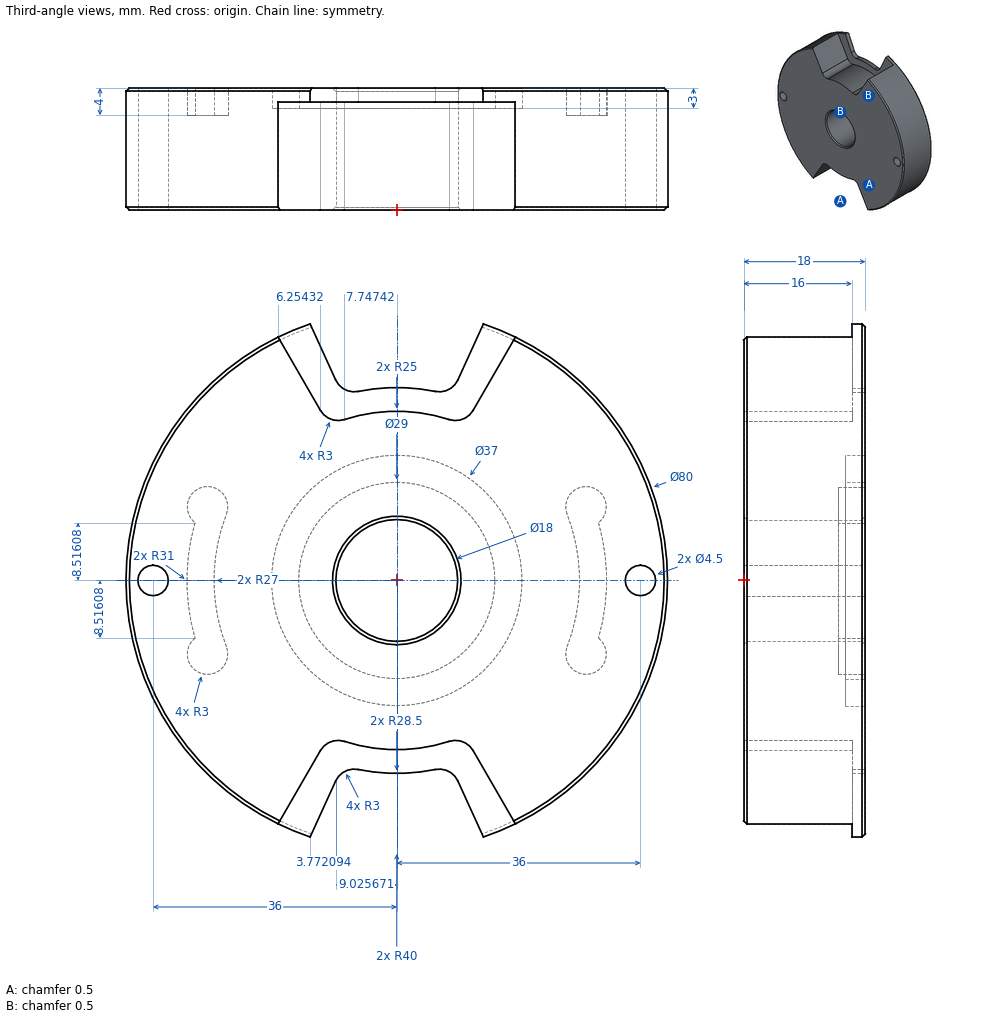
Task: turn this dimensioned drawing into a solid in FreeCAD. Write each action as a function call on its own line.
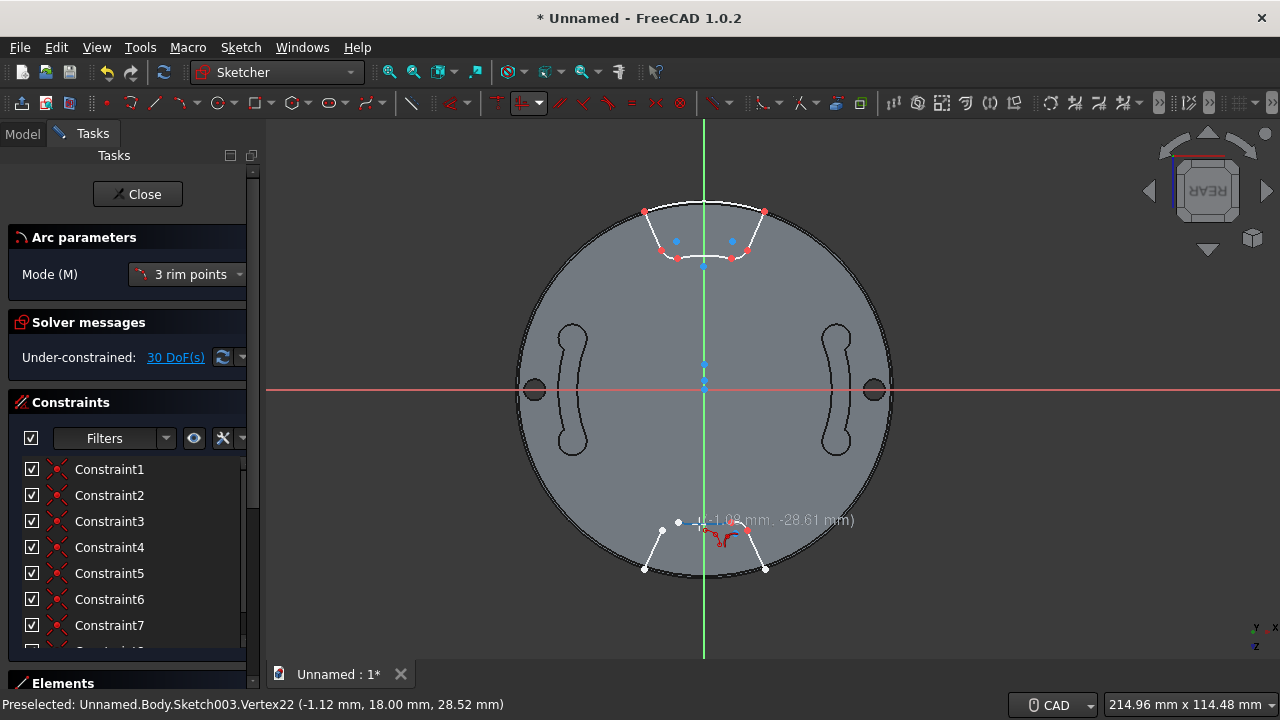
click(678, 523)
click(662, 531)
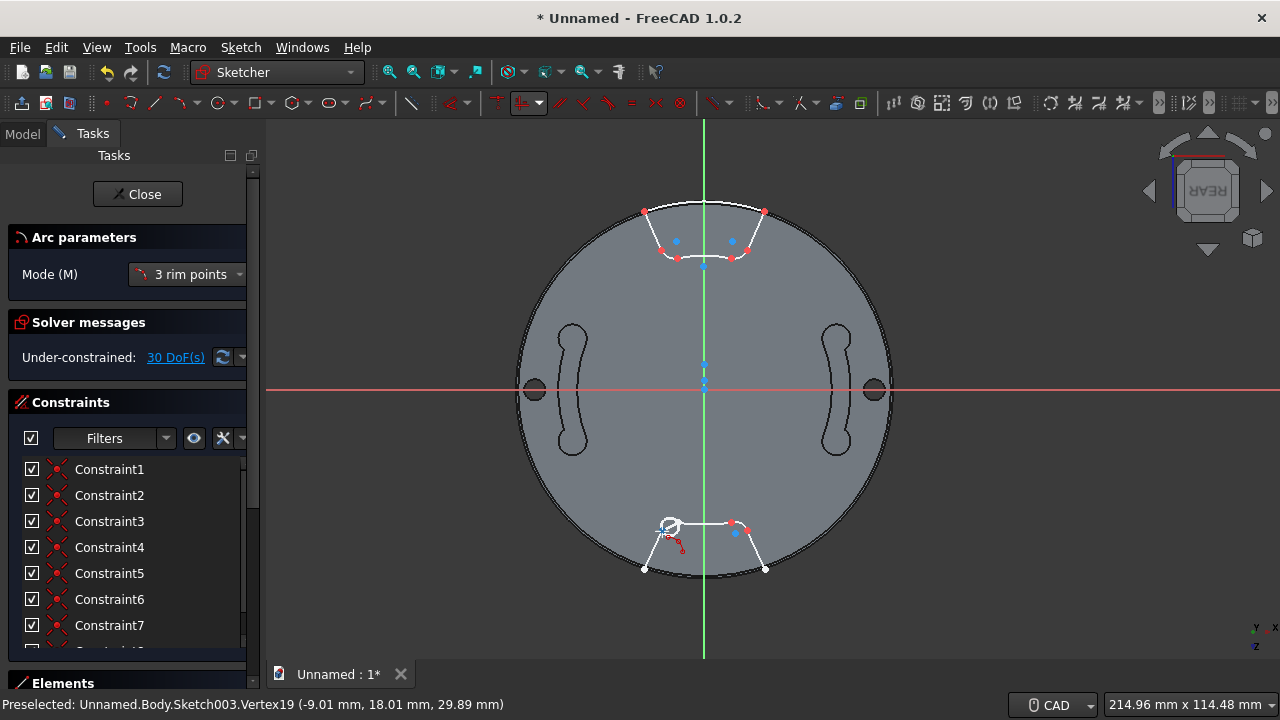
scroll(668, 523, up, 9)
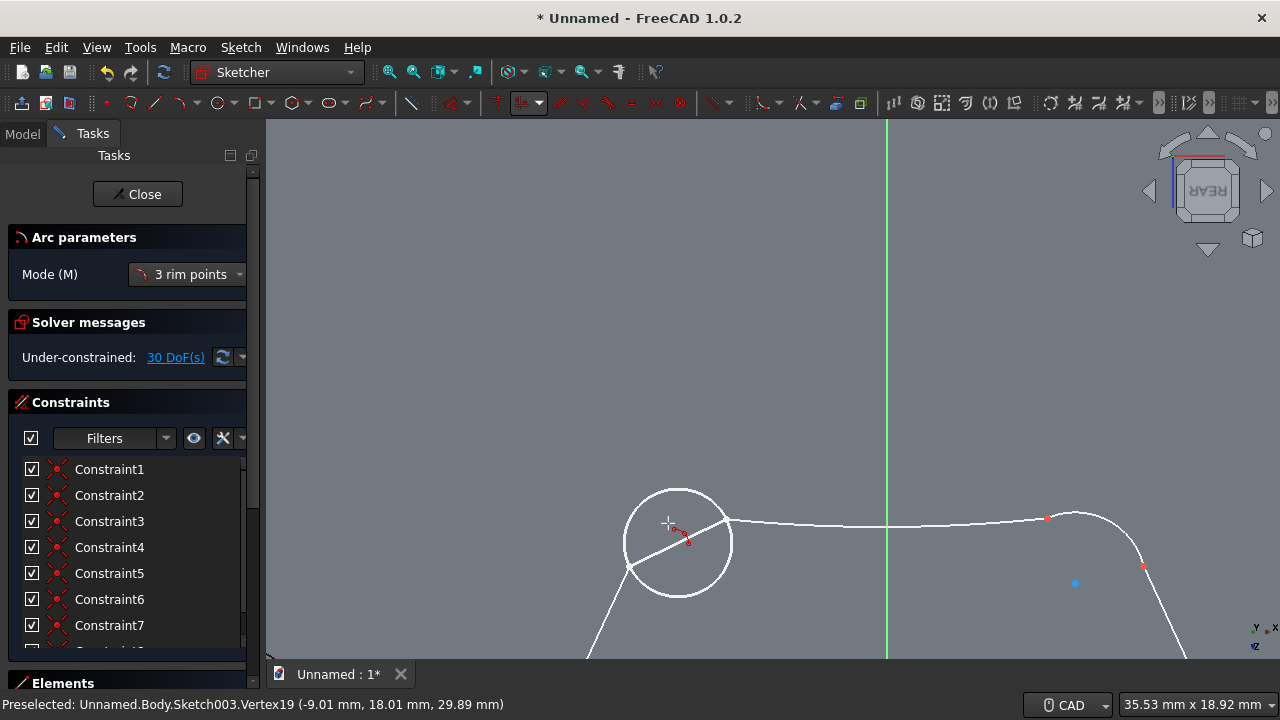
click(668, 518)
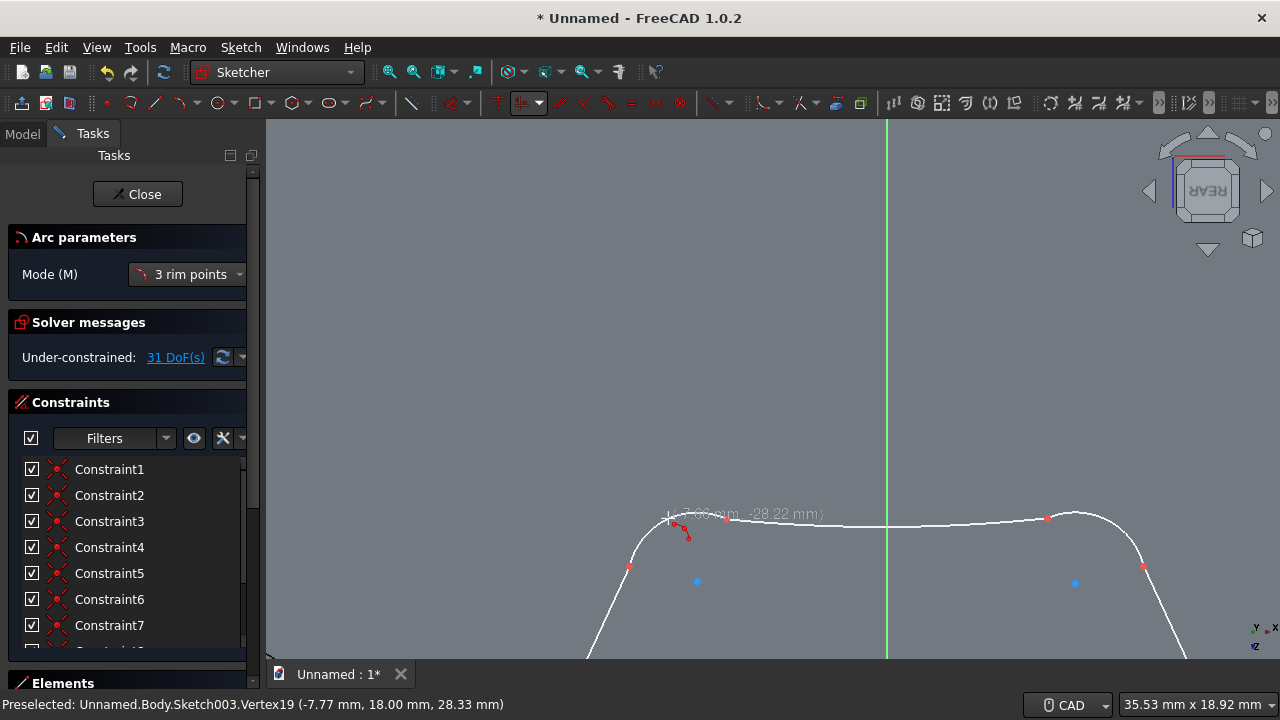
scroll(668, 523, down, 9)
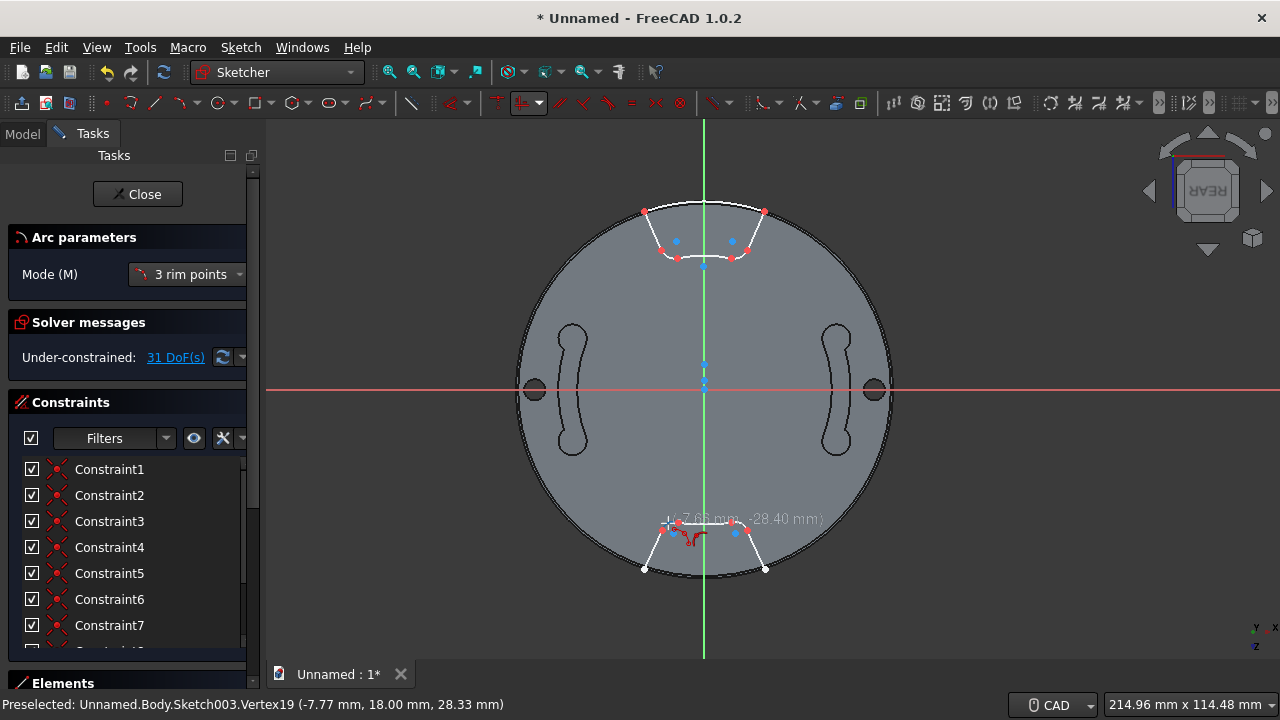
click(644, 570)
click(765, 570)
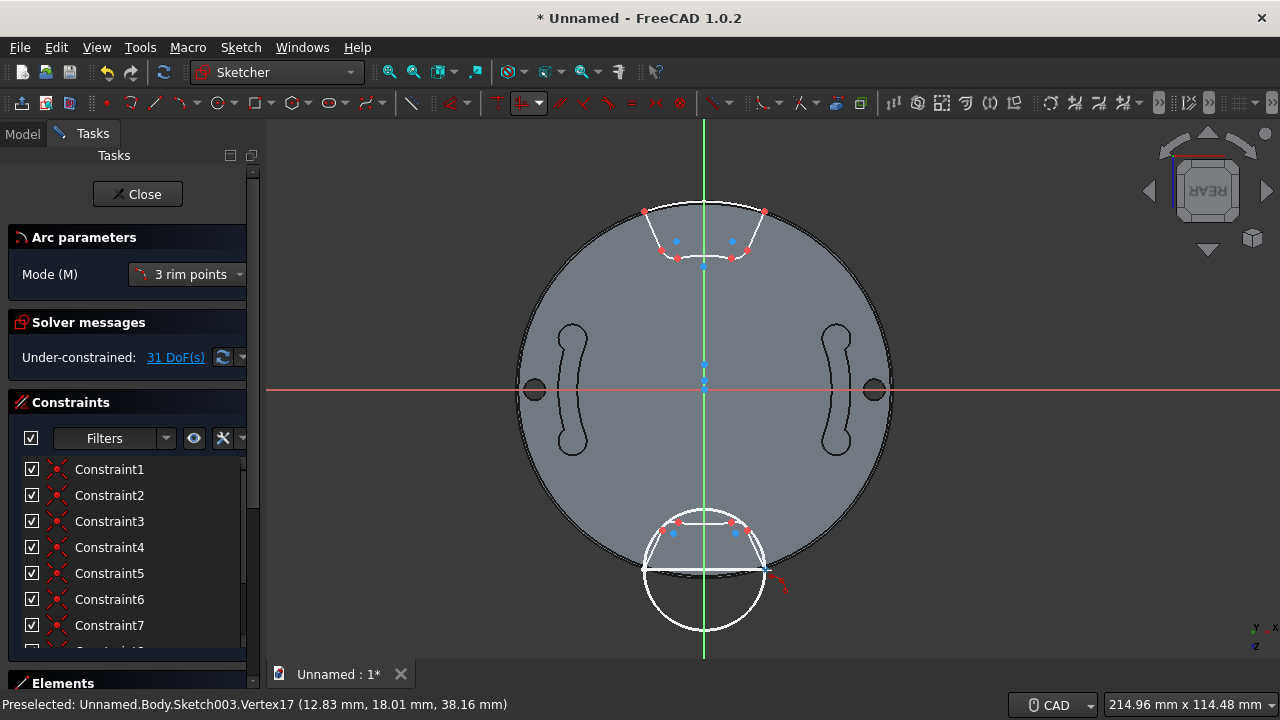
scroll(692, 578, up, 3)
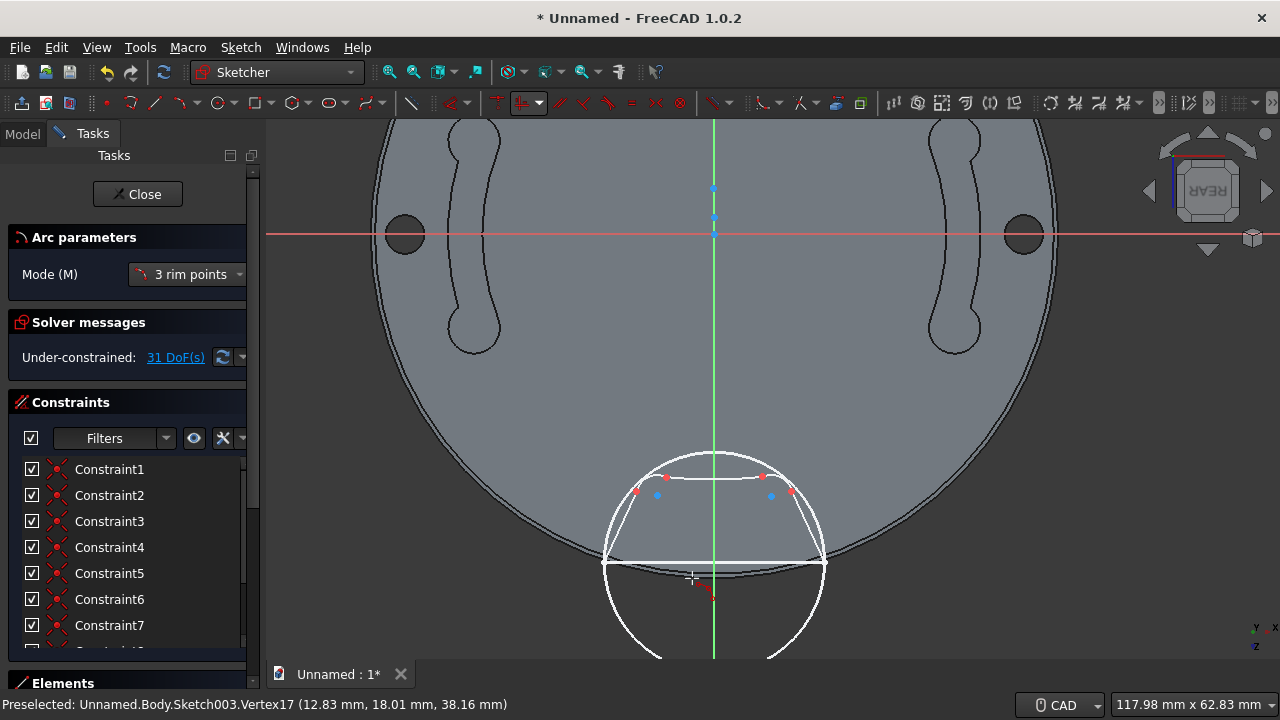
click(692, 578)
key(Escape)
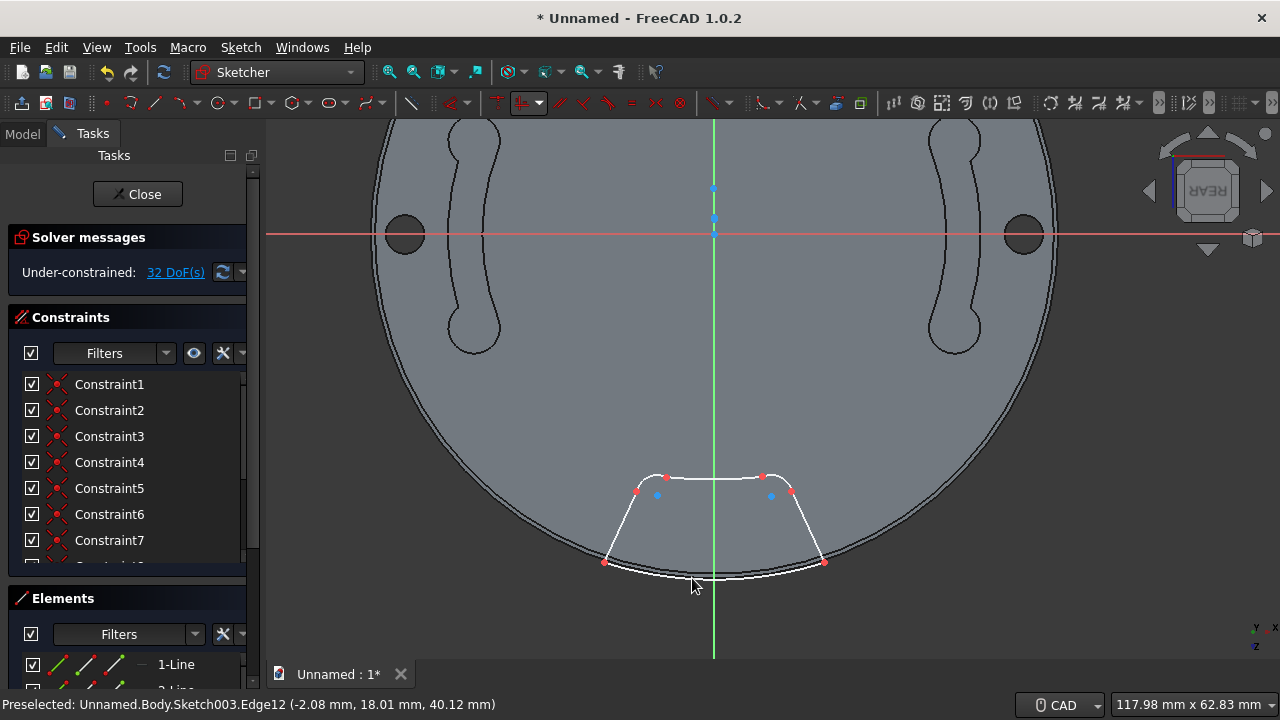
scroll(692, 577, down, 3)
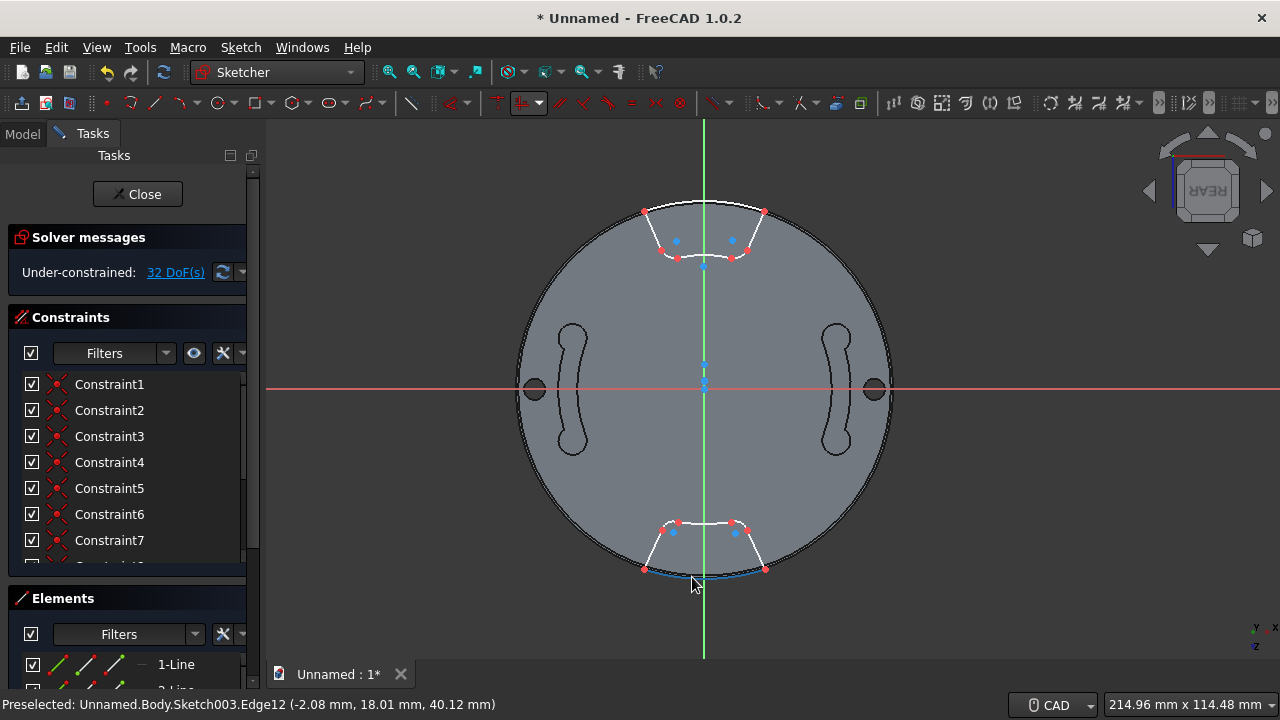
click(650, 223)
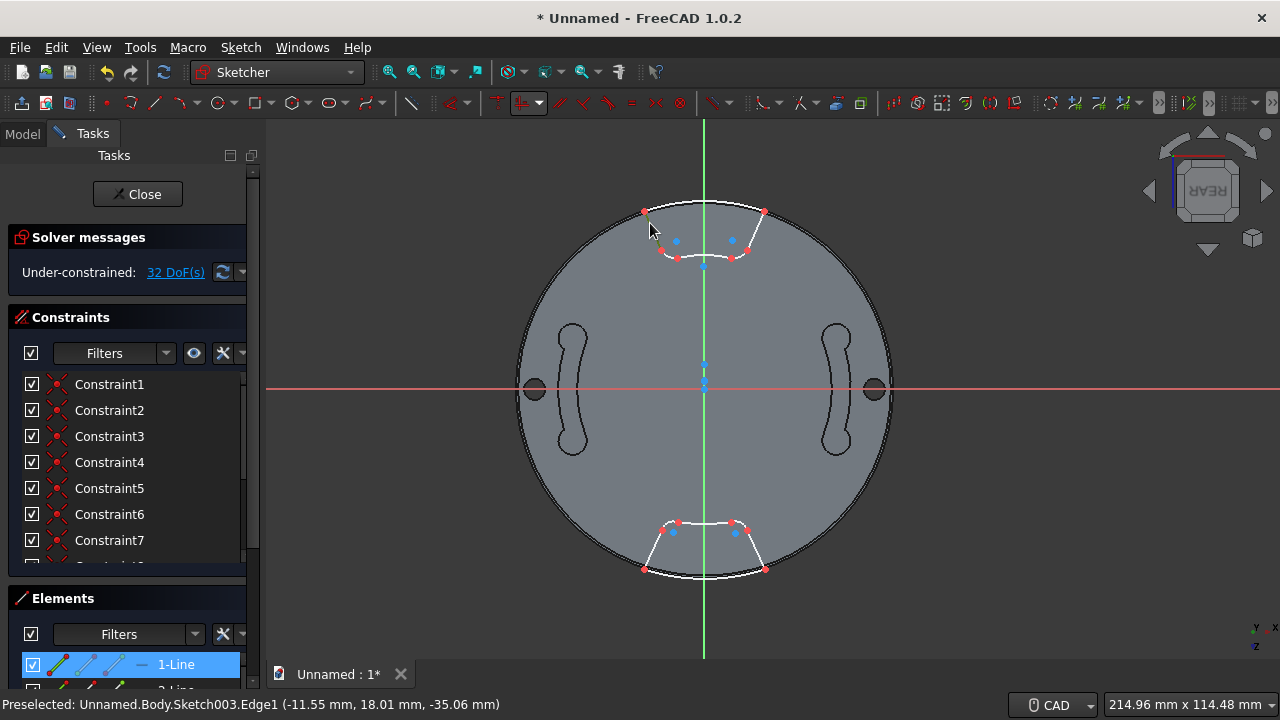
scroll(668, 257, up, 2)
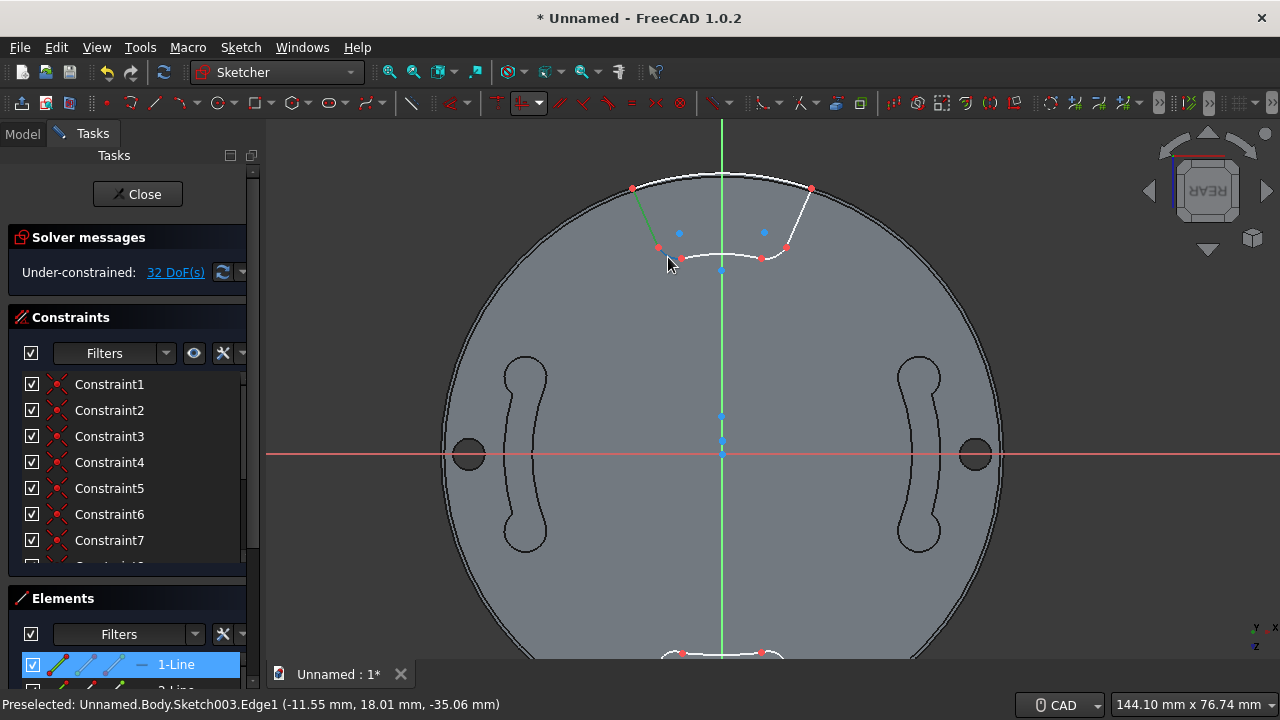
click(668, 256)